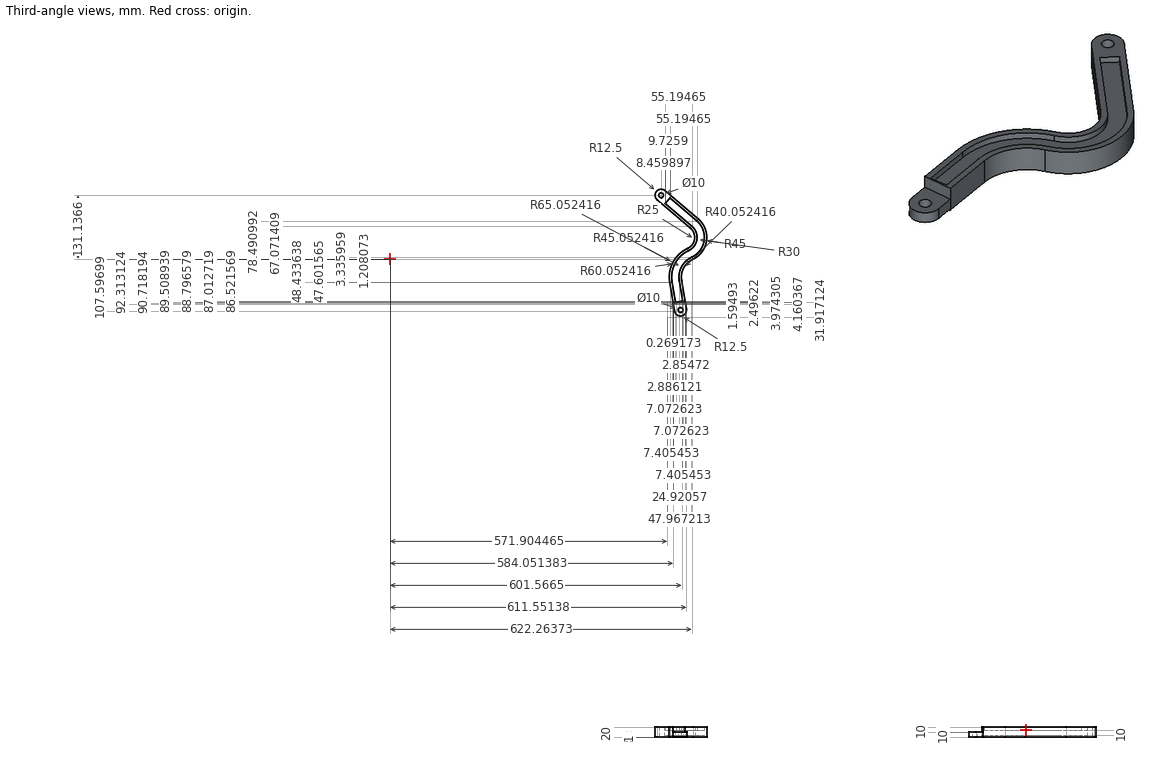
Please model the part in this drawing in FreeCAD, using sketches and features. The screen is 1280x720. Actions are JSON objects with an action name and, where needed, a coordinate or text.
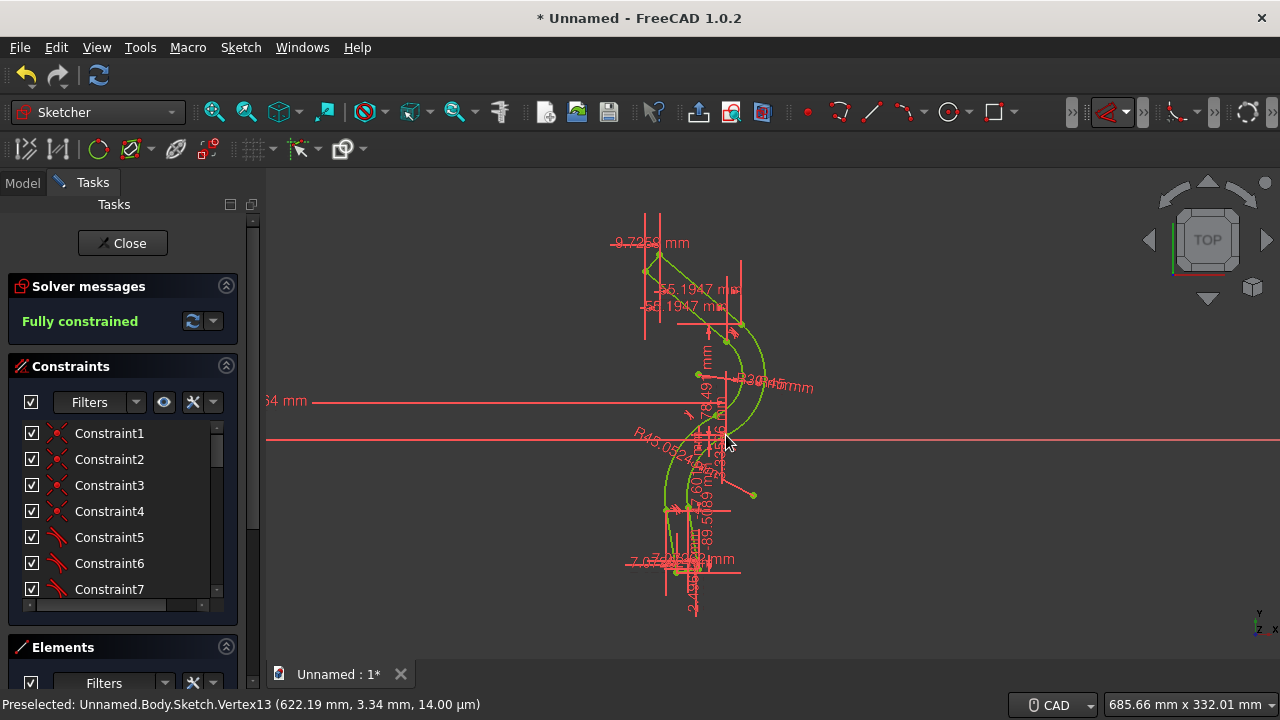
{"action": "left_click", "coordinate": [123, 243]}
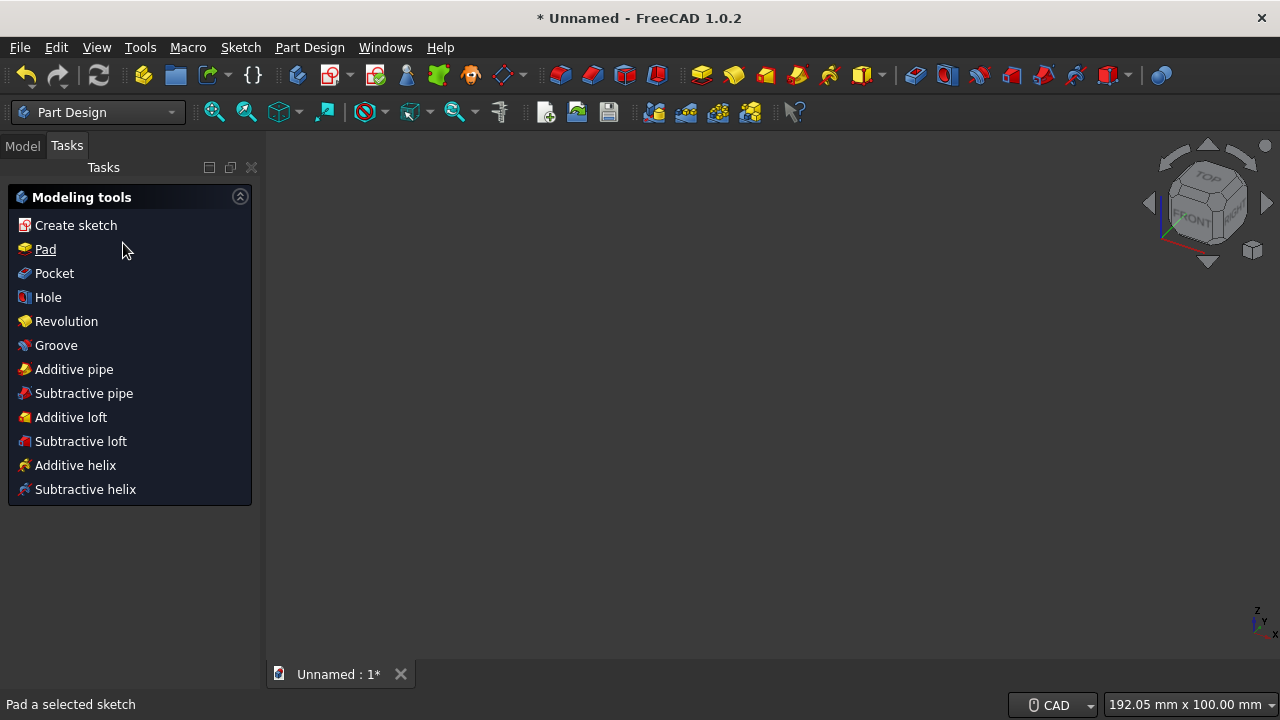
{"action": "left_click", "coordinate": [702, 76]}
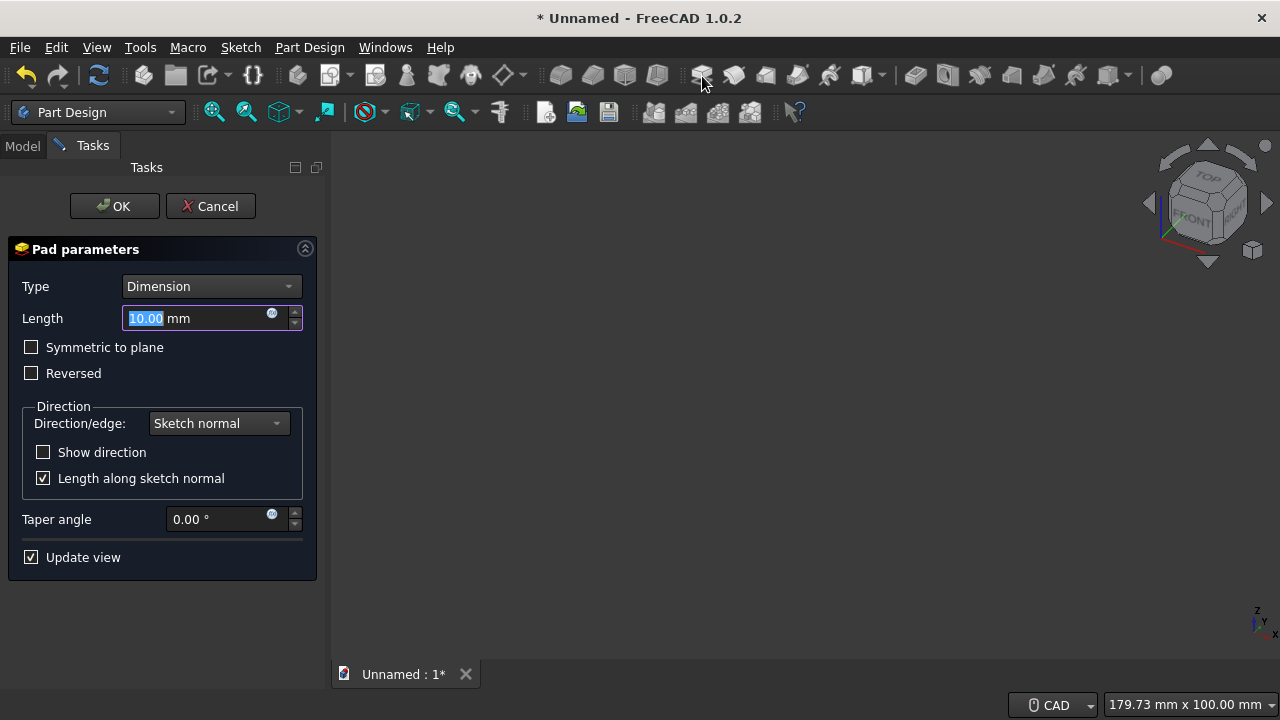
{"action": "type", "text": "10"}
{"action": "key", "text": "Tab"}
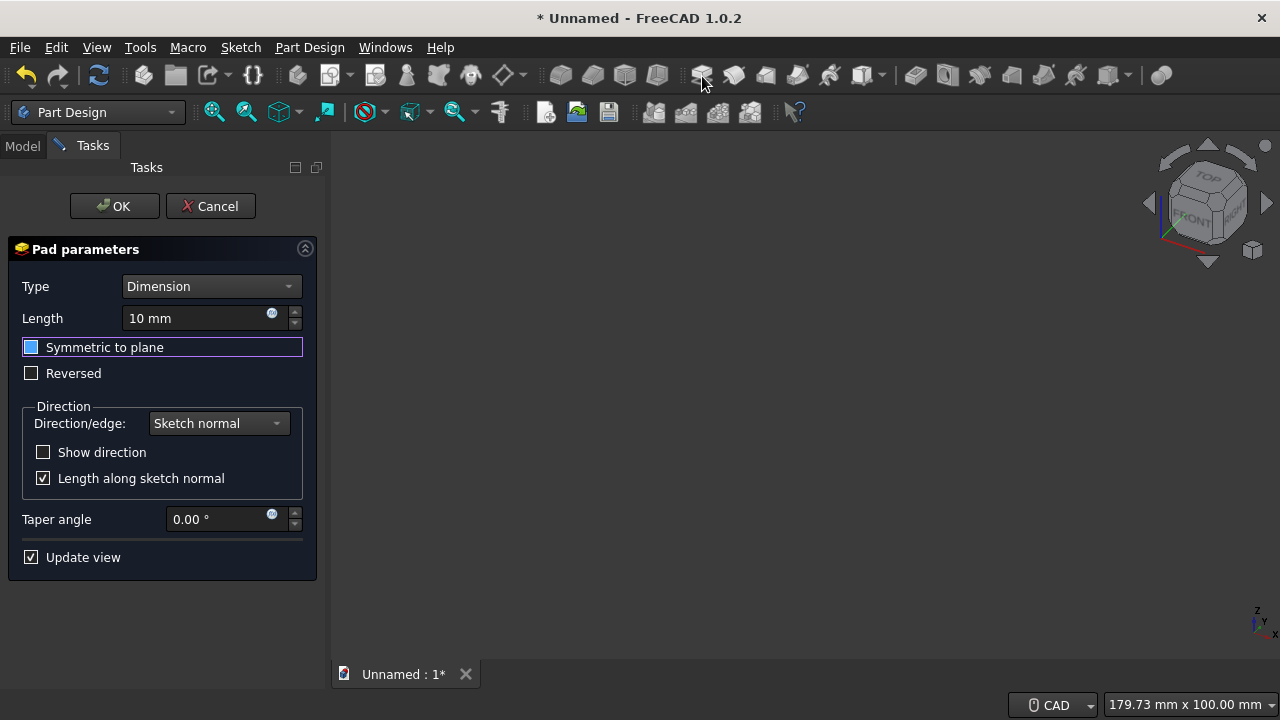
{"action": "left_click", "coordinate": [30, 373]}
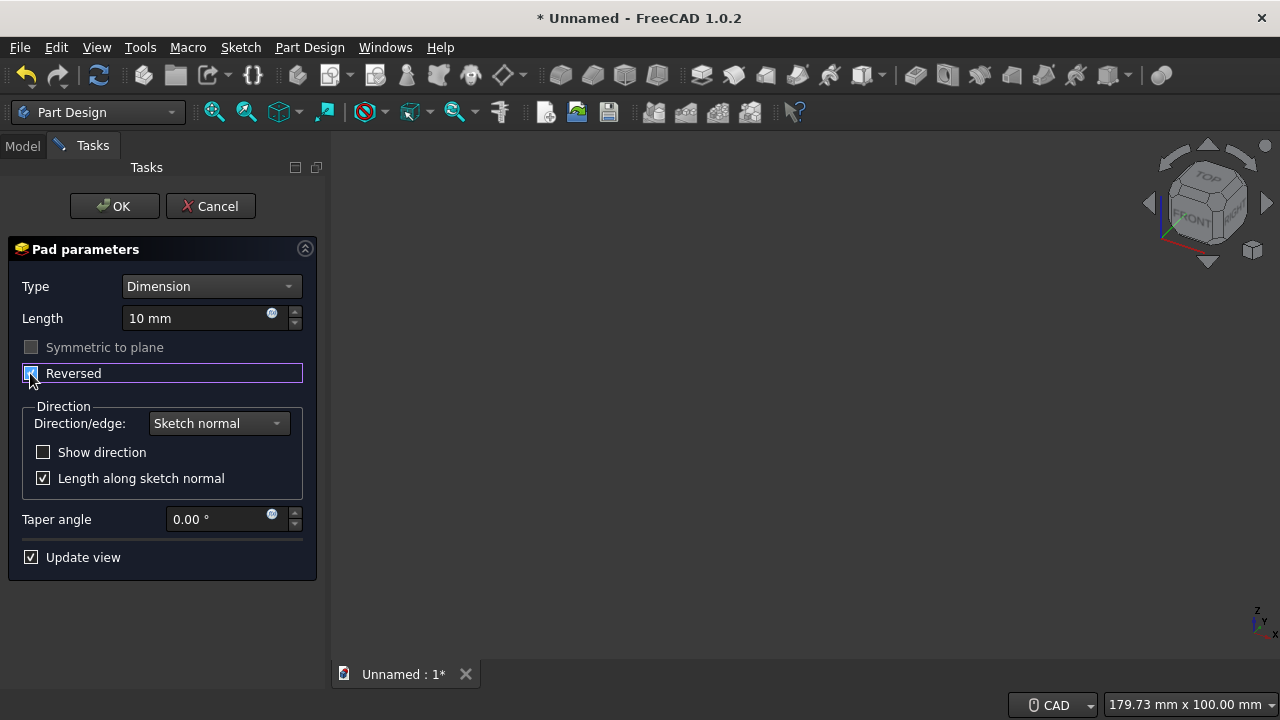
{"action": "left_click", "coordinate": [115, 206]}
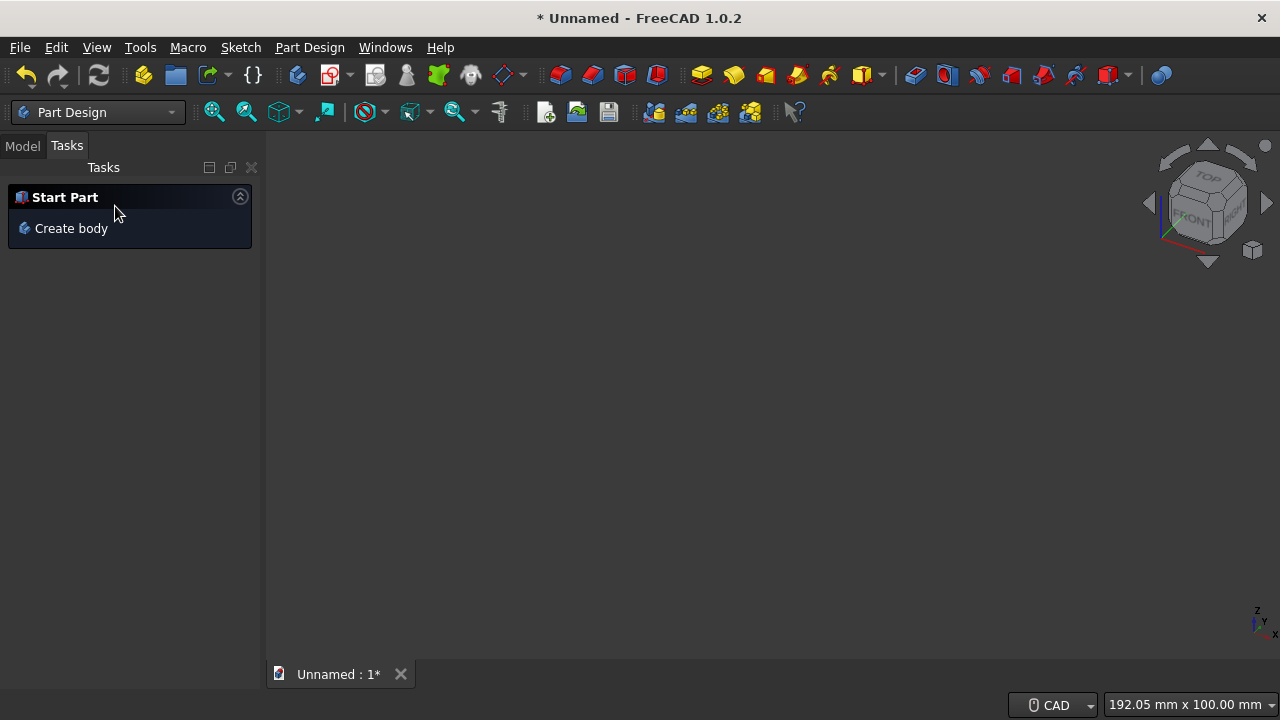
{"action": "key", "text": "v f"}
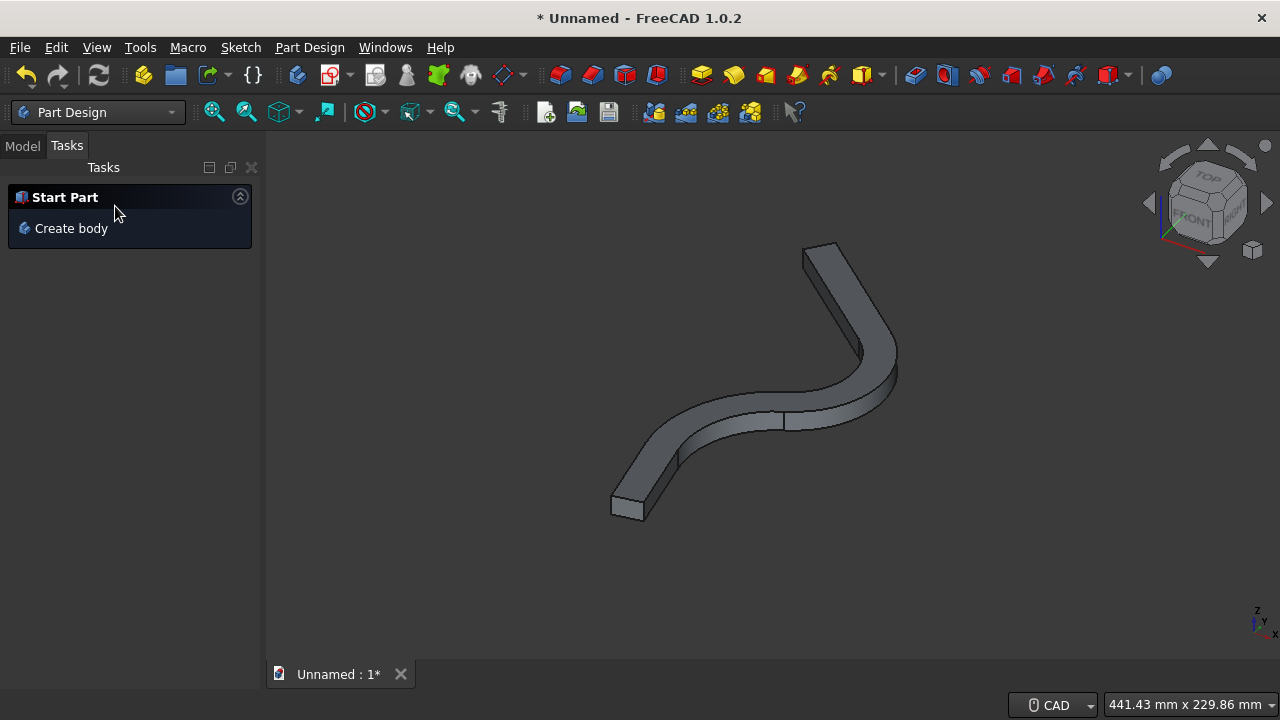
{"action": "left_click", "coordinate": [23, 145]}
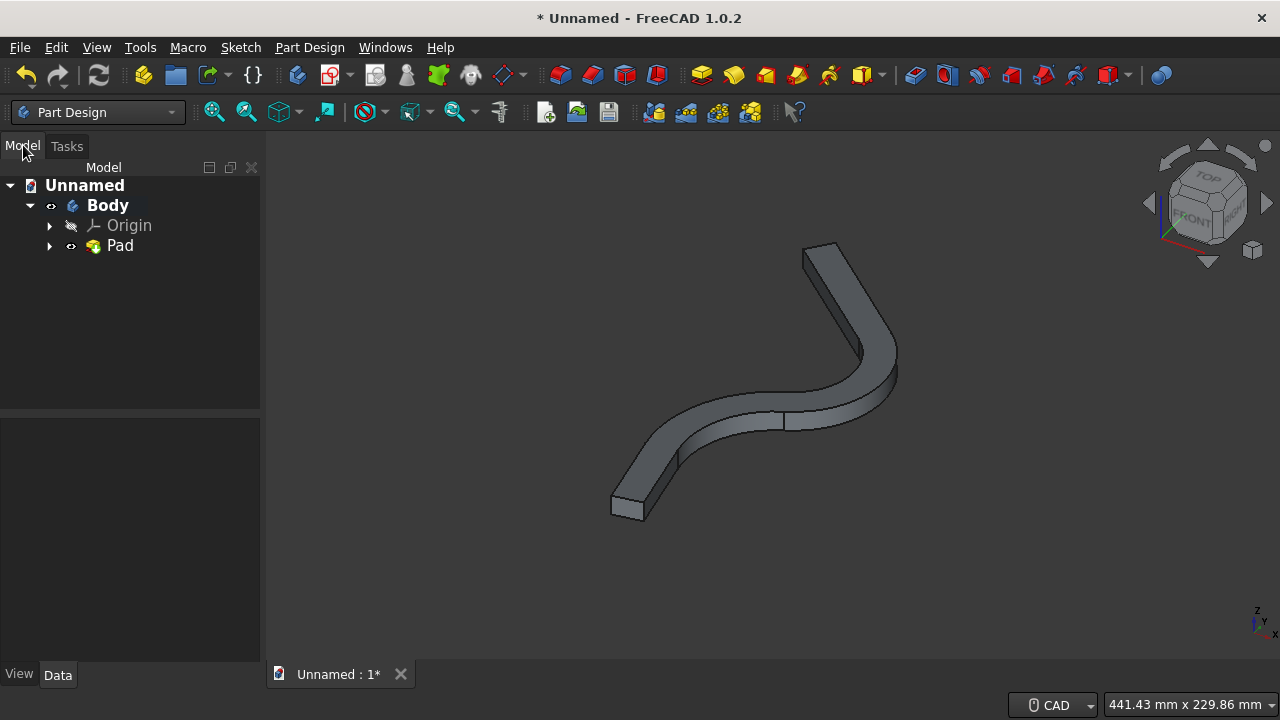
{"action": "left_click", "coordinate": [50, 226]}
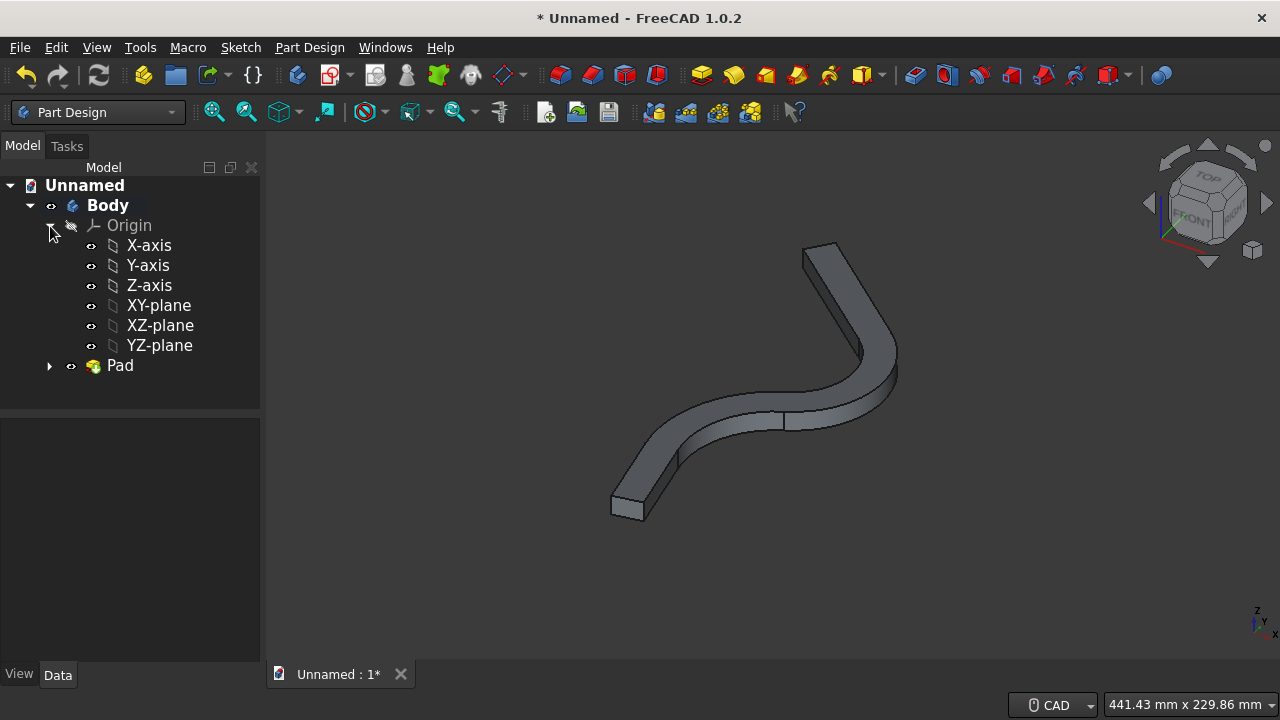
{"action": "left_click", "coordinate": [136, 306]}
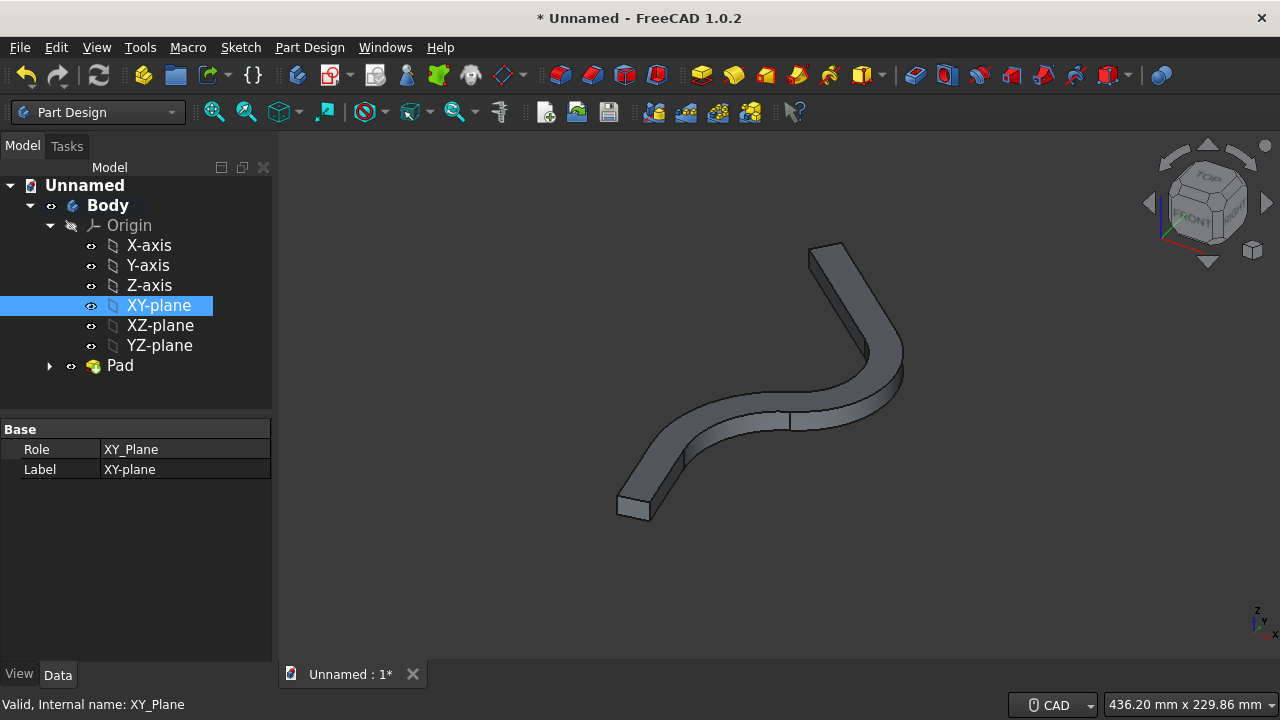
{"action": "left_click", "coordinate": [504, 76]}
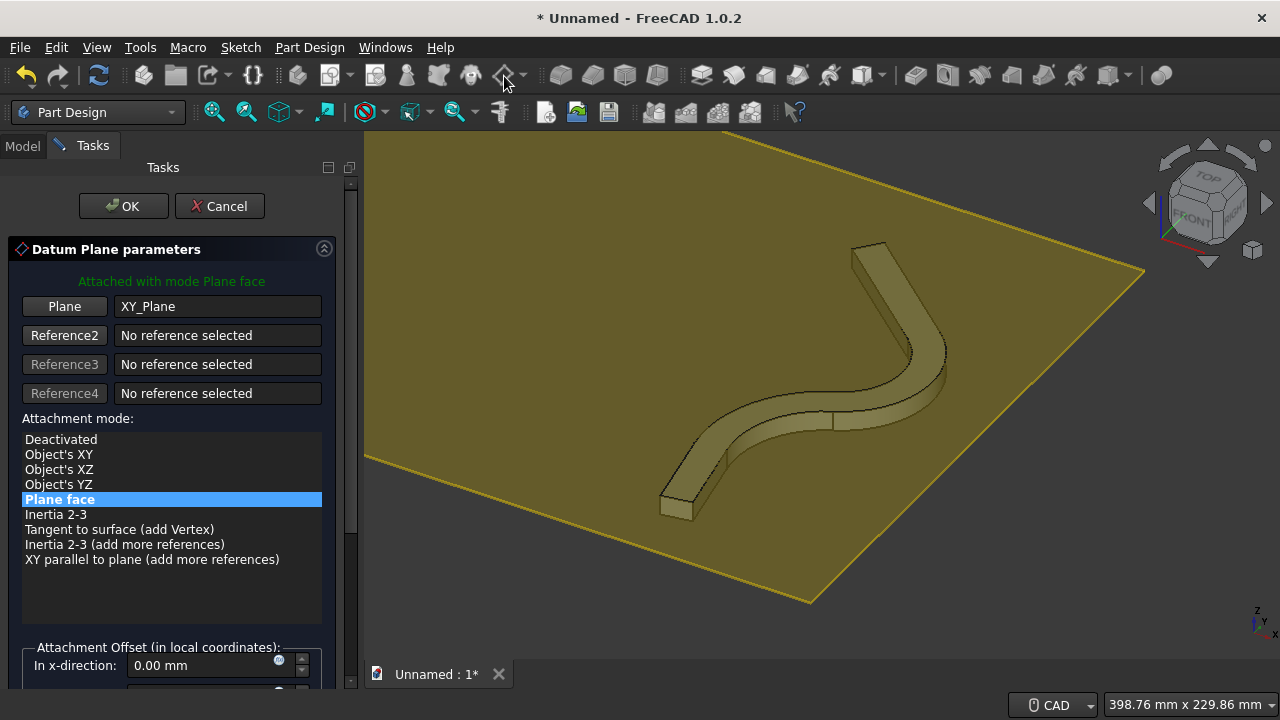
{"action": "scroll", "coordinate": [351, 432], "scroll_direction": "down", "scroll_amount": 2}